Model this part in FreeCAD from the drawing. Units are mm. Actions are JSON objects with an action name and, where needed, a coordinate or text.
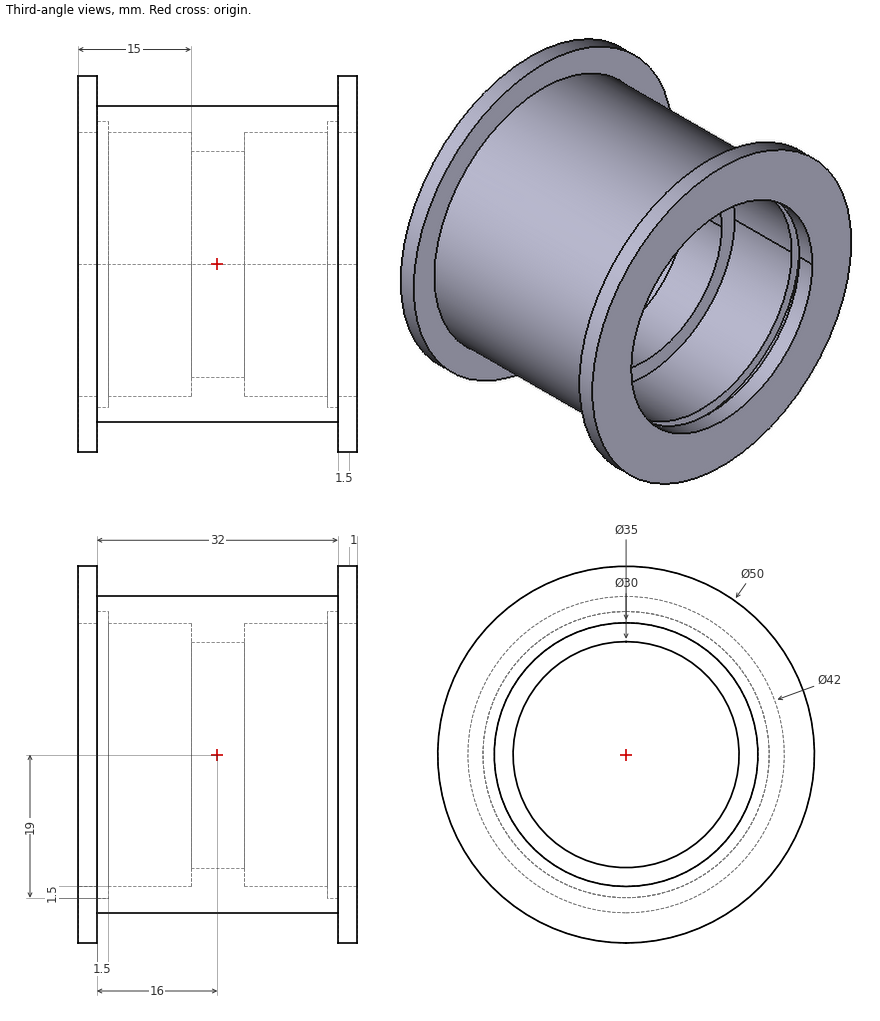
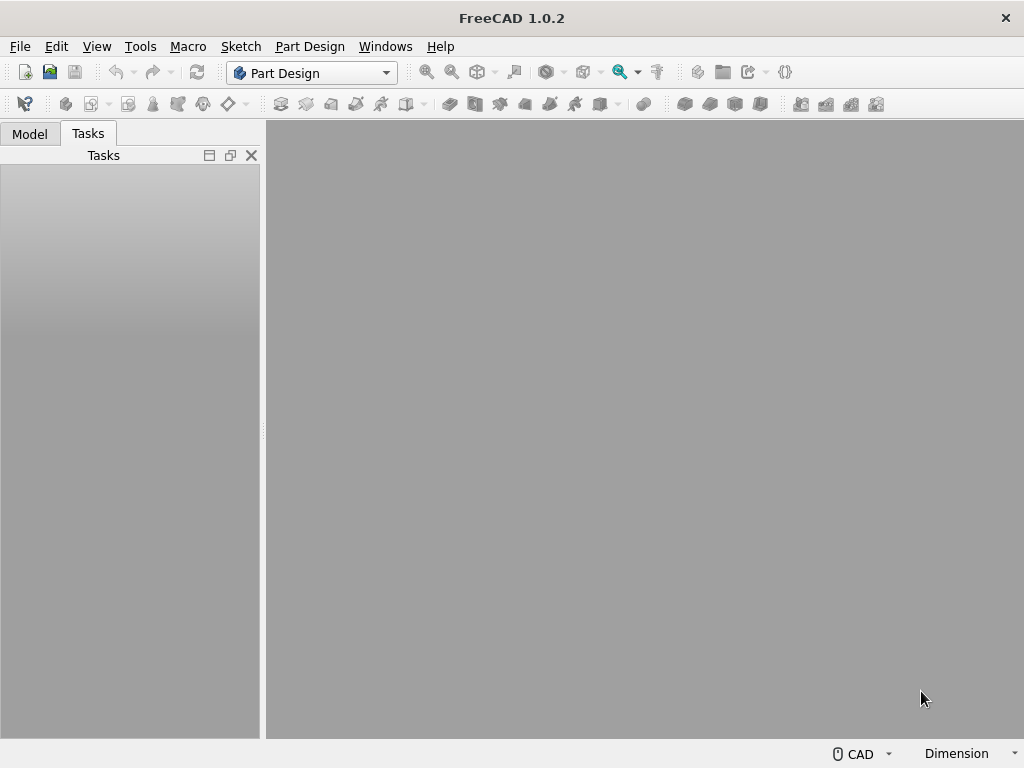
{"action": "left_click", "coordinate": [25, 72]}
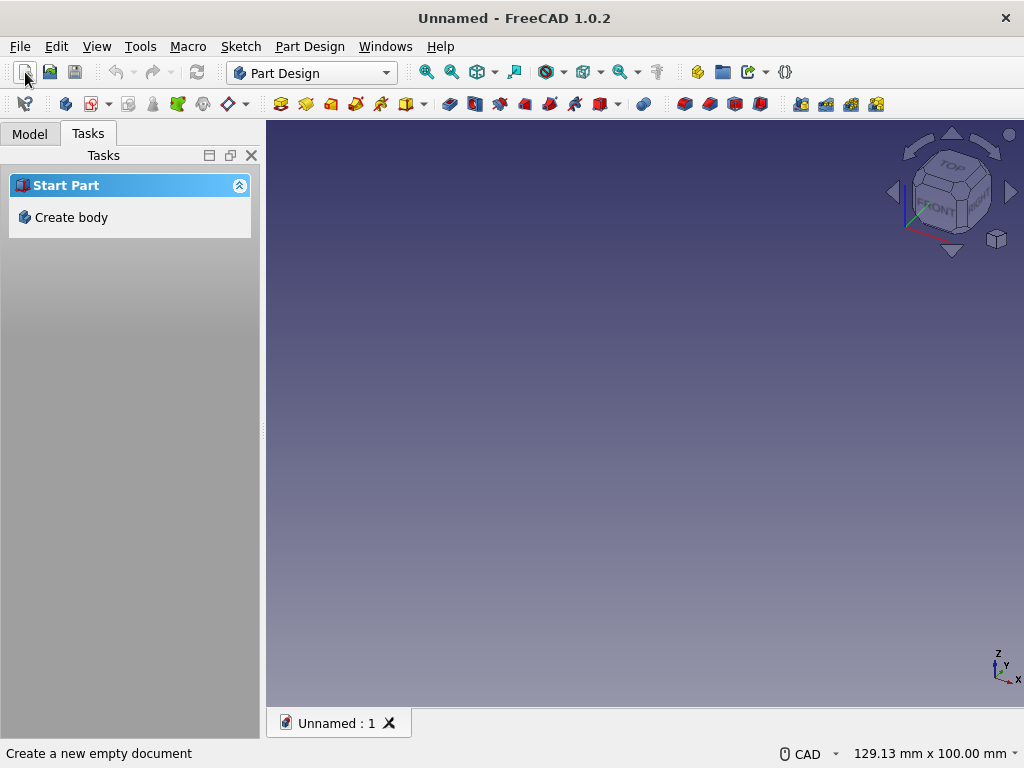
{"action": "left_click", "coordinate": [90, 104]}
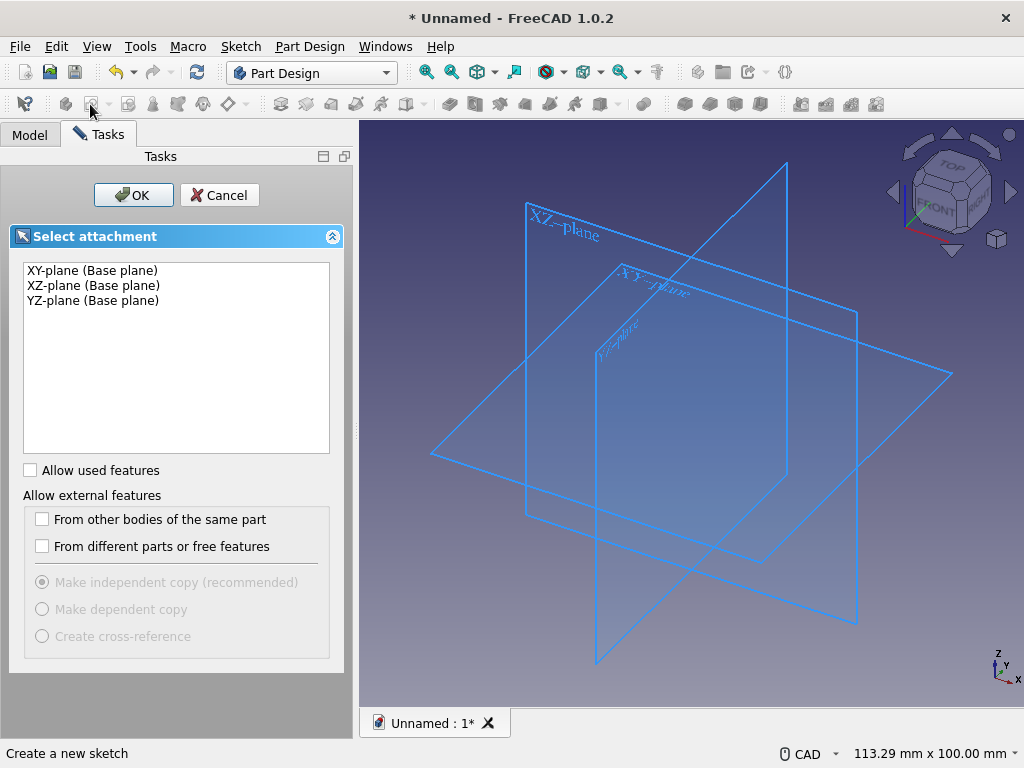
{"action": "left_click", "coordinate": [84, 300]}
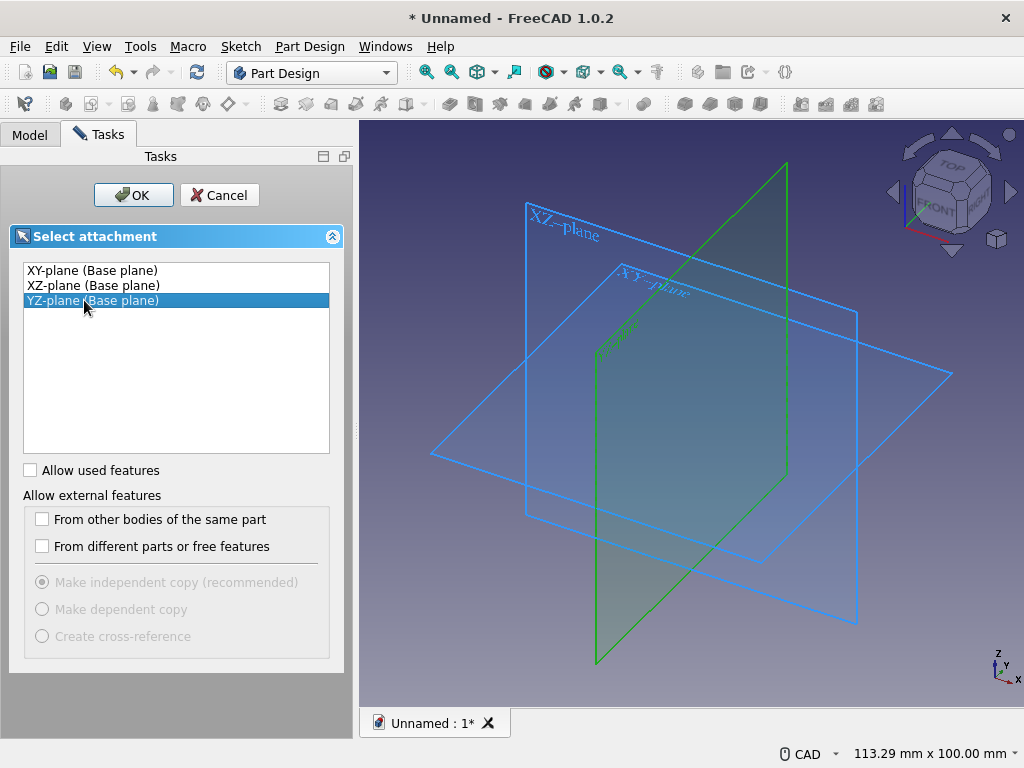
{"action": "left_click", "coordinate": [134, 195]}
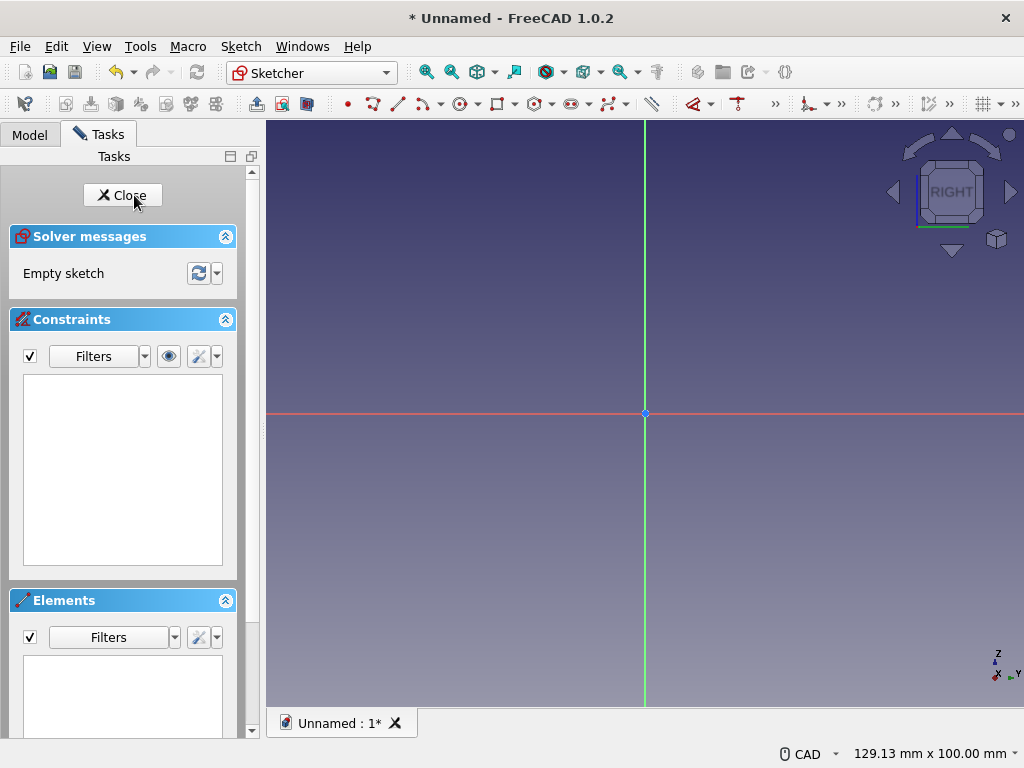
{"action": "scroll", "coordinate": [784, 413], "scroll_direction": "up", "scroll_amount": 2}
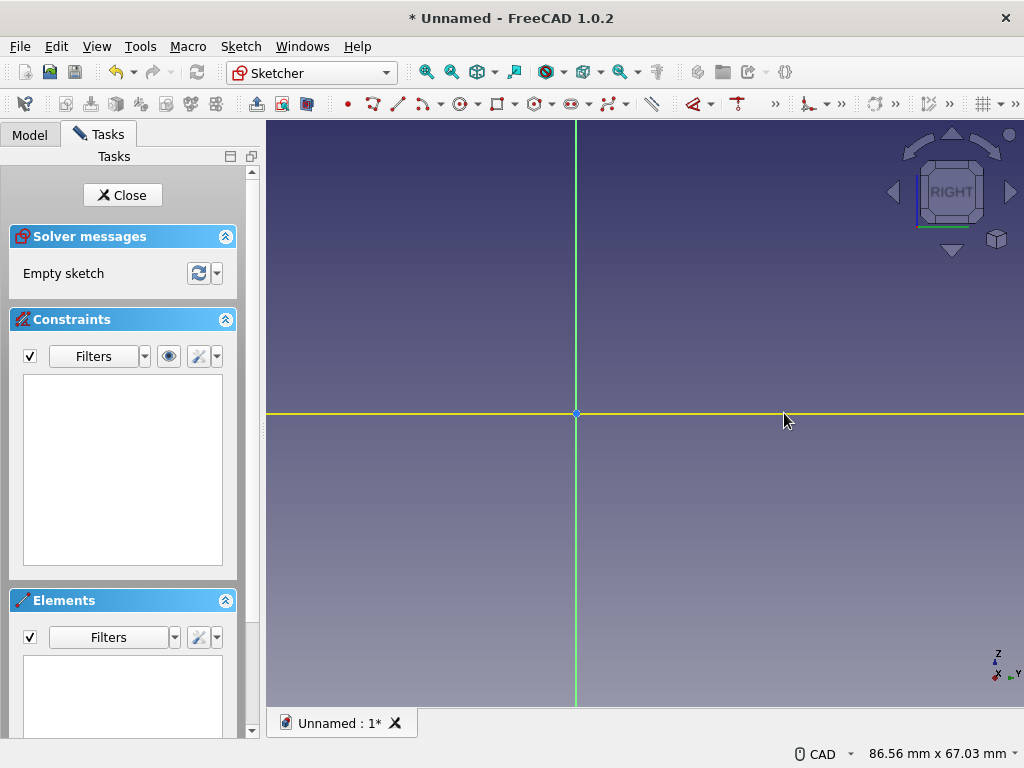
{"action": "key", "text": "g c"}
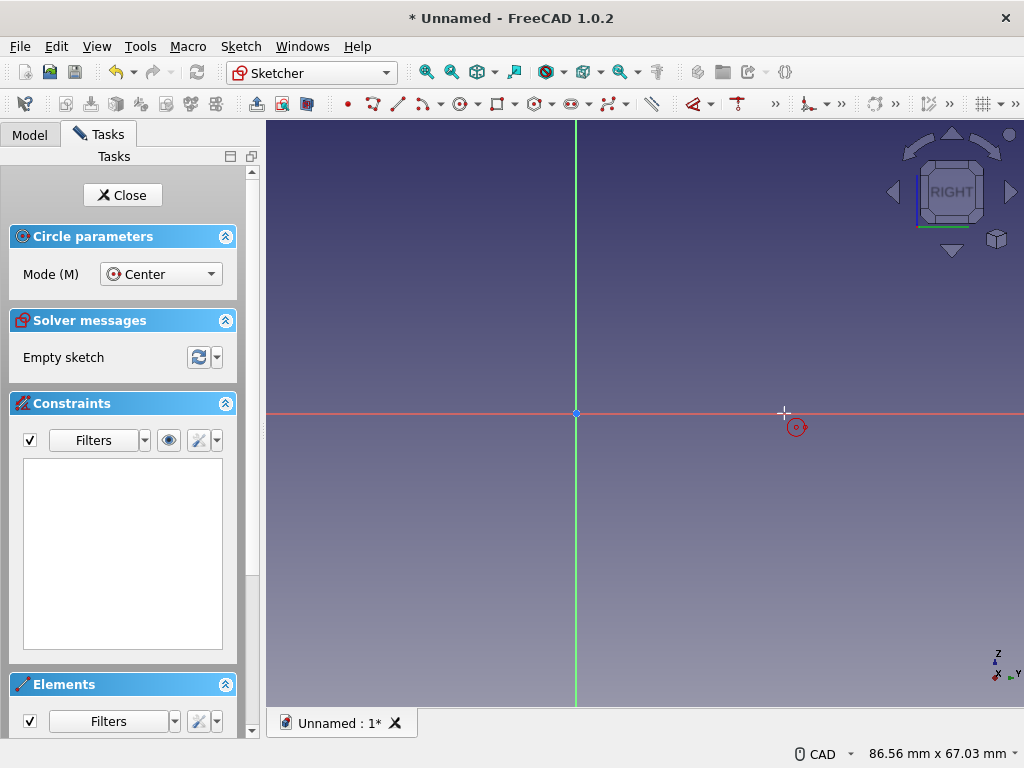
{"action": "left_click", "coordinate": [576, 414]}
{"action": "mouse_move", "coordinate": [706, 283]}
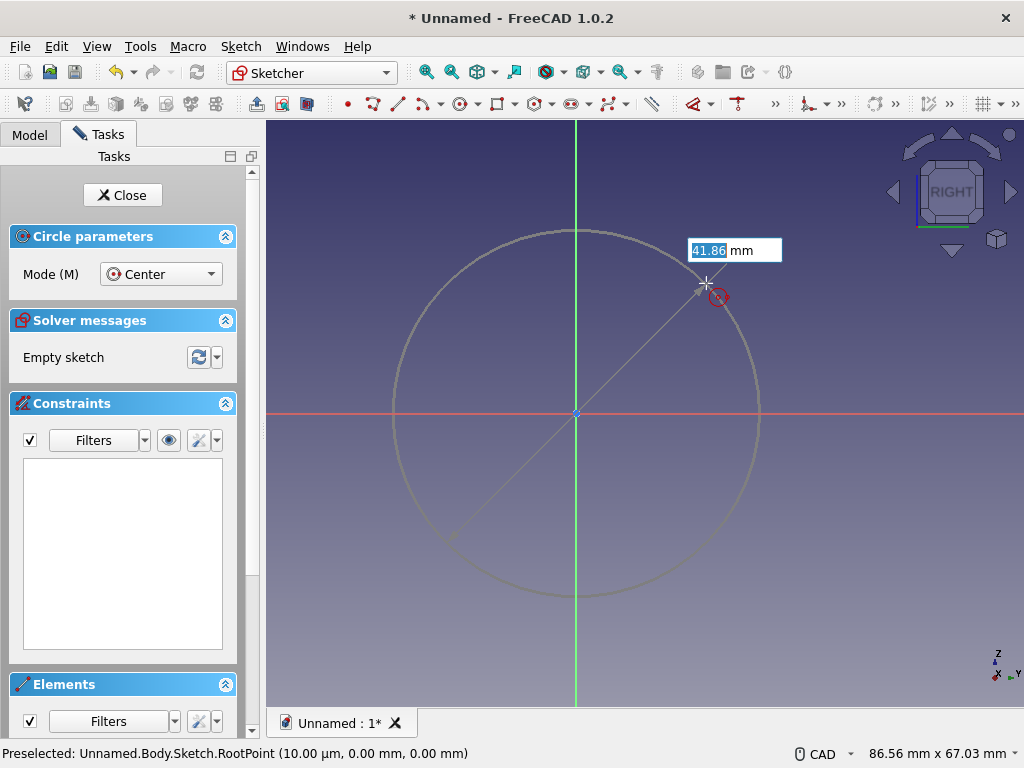
{"action": "type", "text": "42"}
{"action": "key", "text": "Return"}
{"action": "key", "text": "Escape"}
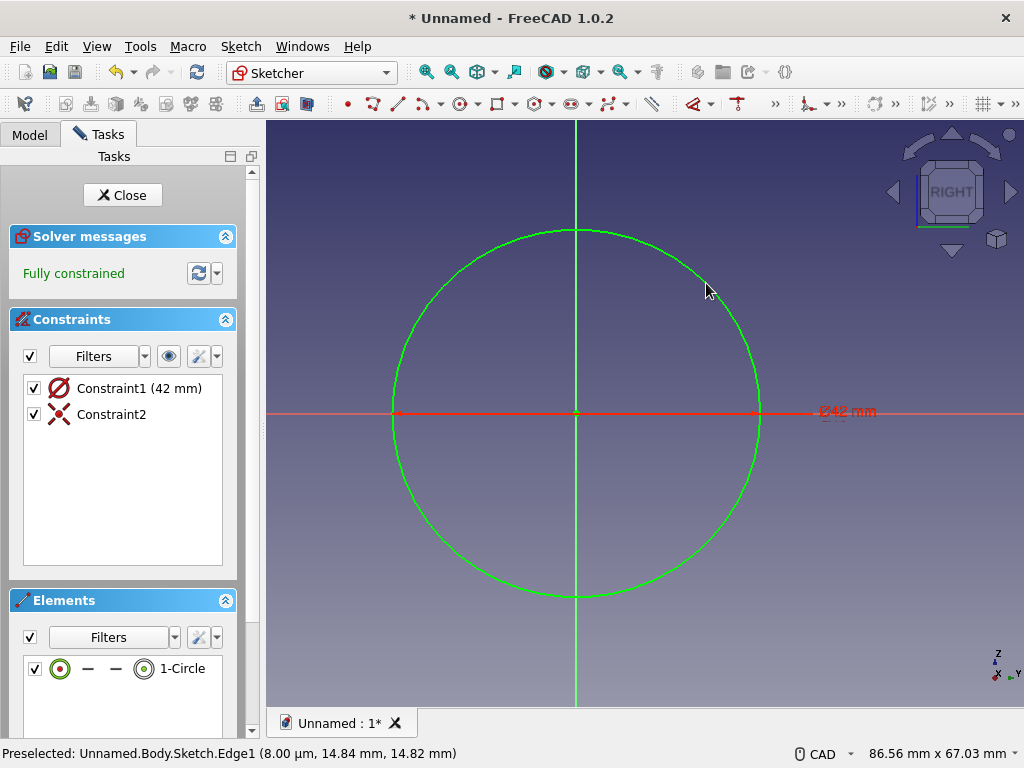
{"action": "left_click", "coordinate": [123, 195]}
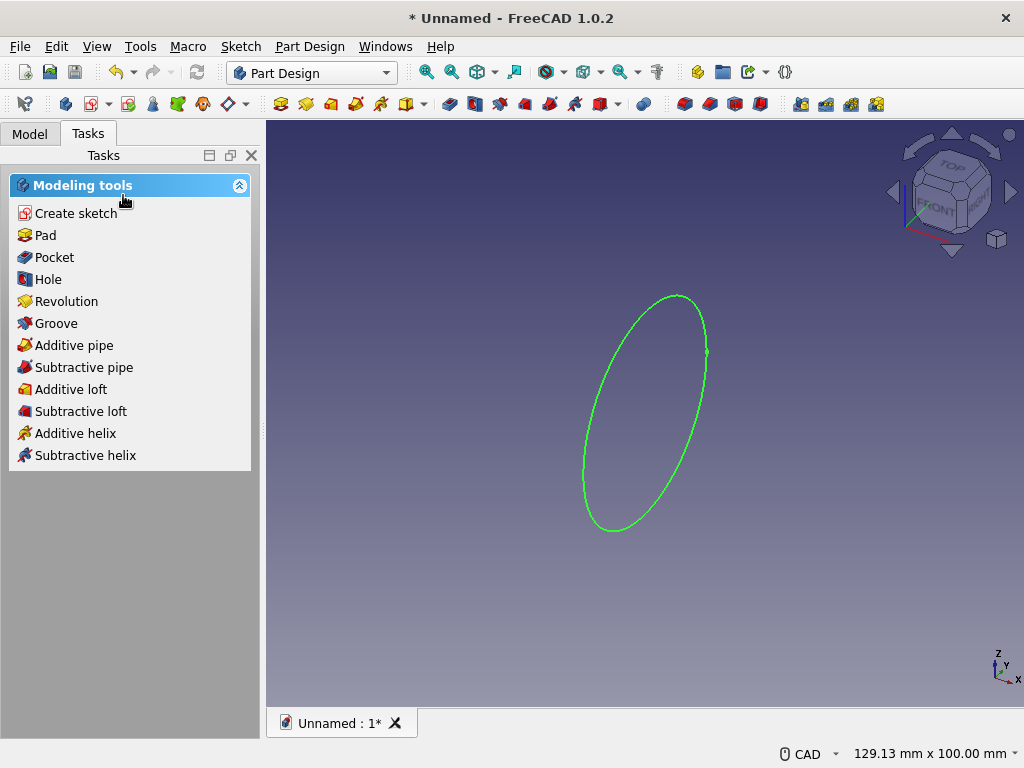
{"action": "left_click", "coordinate": [281, 104]}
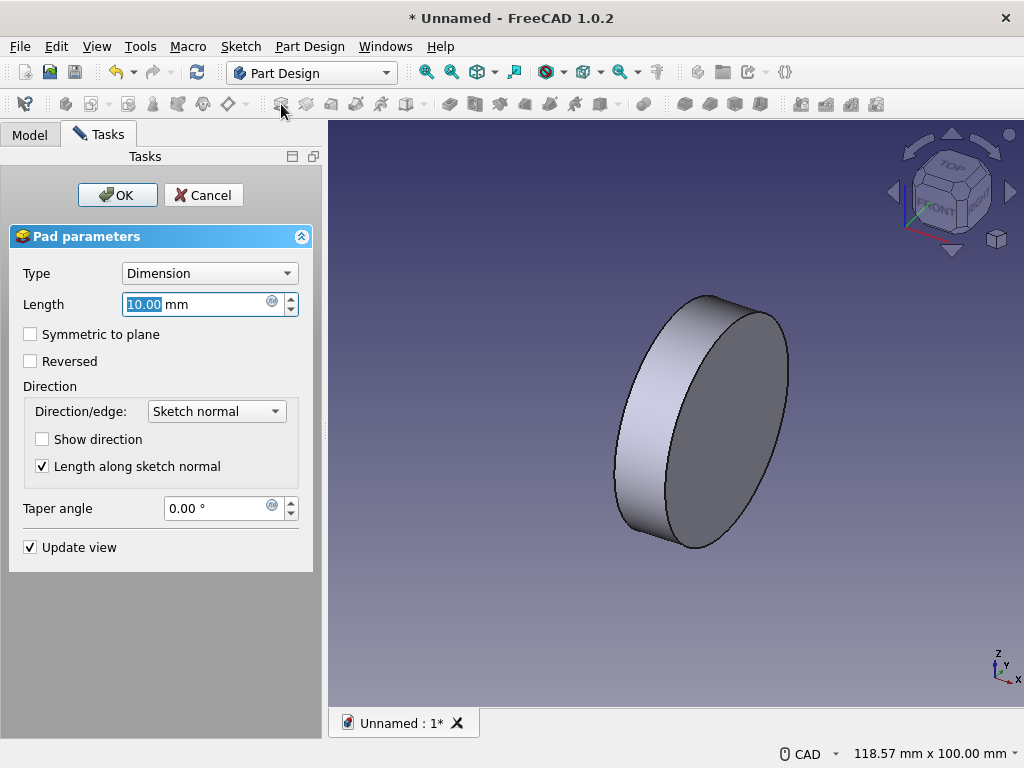
{"action": "type", "text": "32"}
{"action": "key", "text": "Tab"}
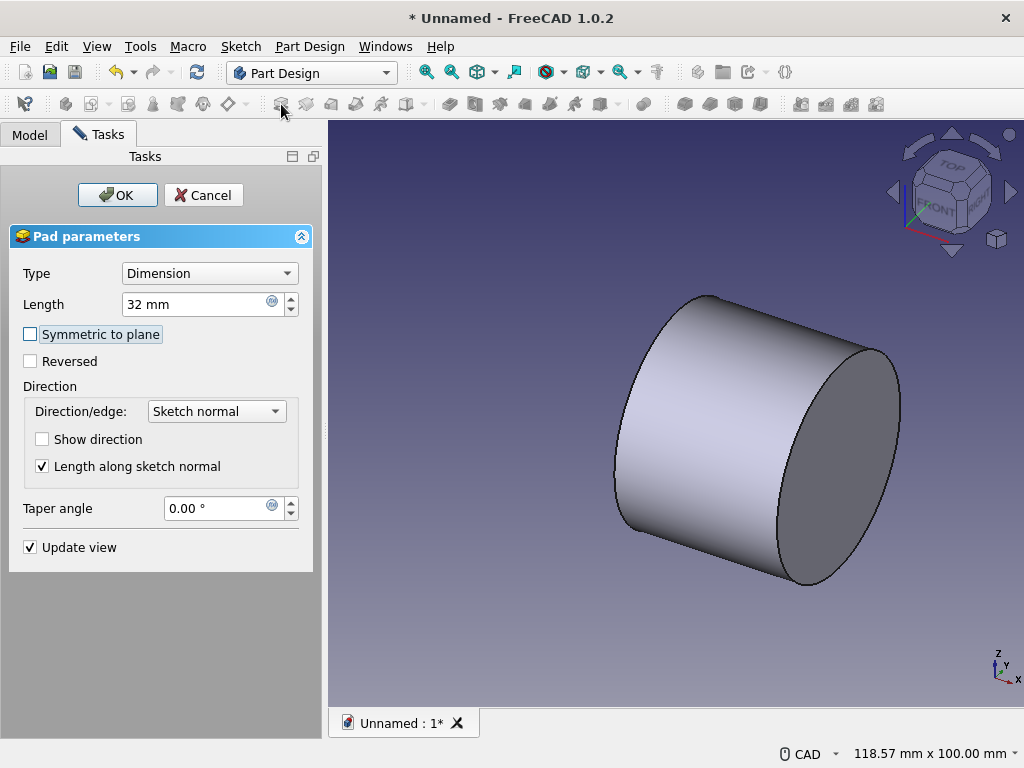
{"action": "left_click", "coordinate": [31, 334]}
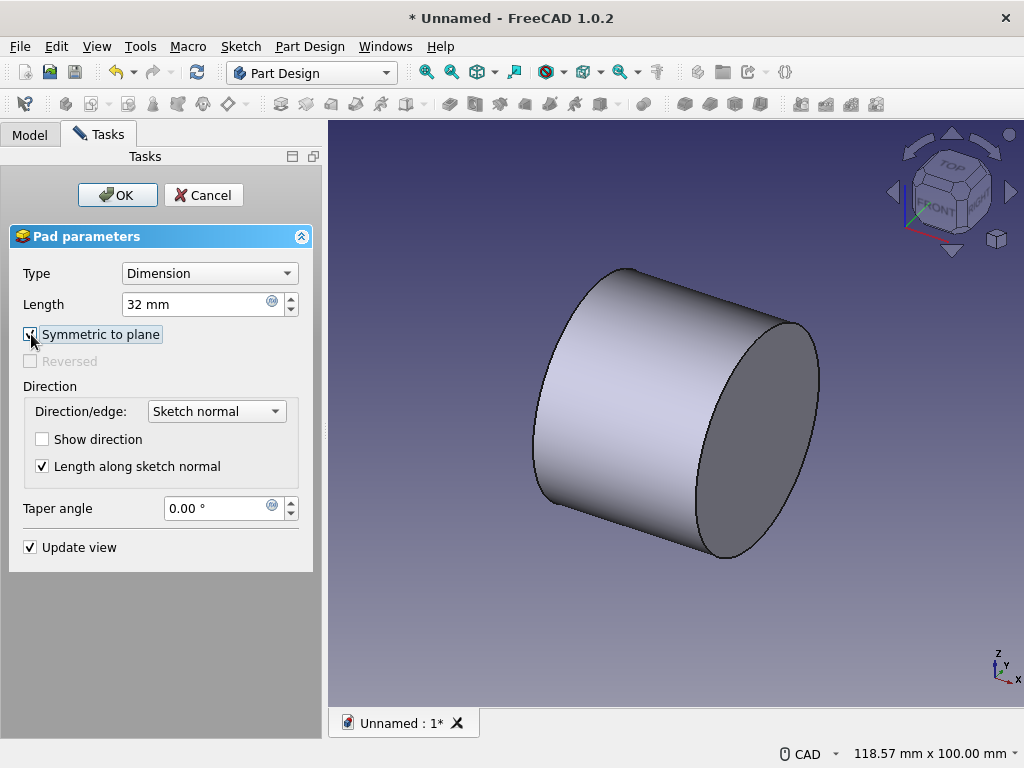
{"action": "left_click", "coordinate": [118, 195]}